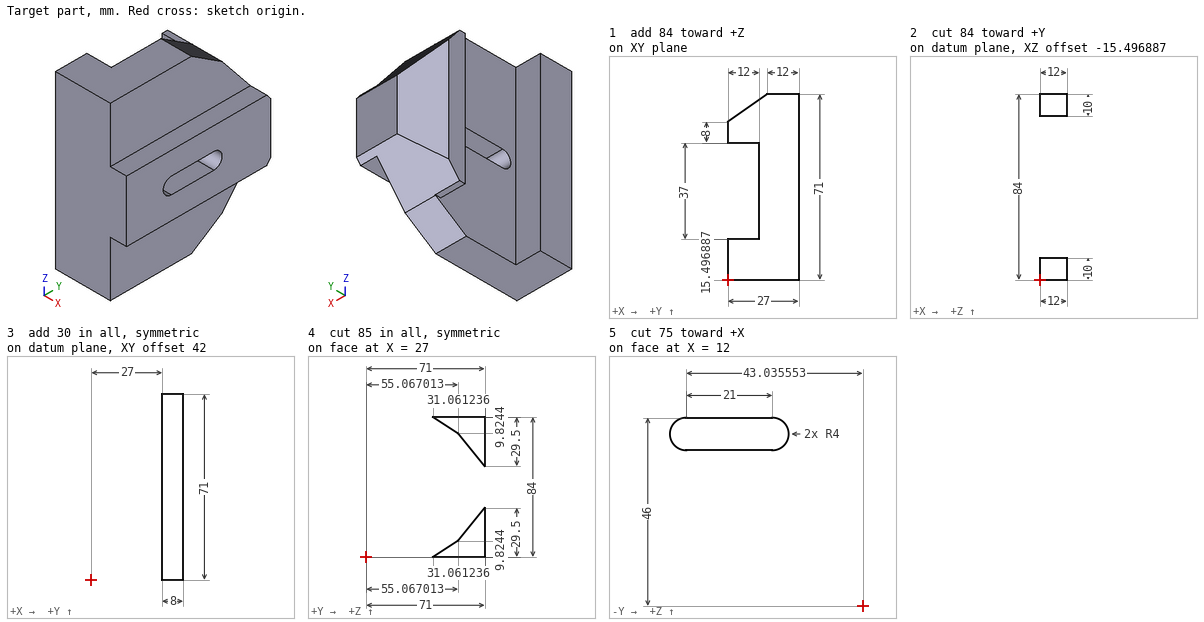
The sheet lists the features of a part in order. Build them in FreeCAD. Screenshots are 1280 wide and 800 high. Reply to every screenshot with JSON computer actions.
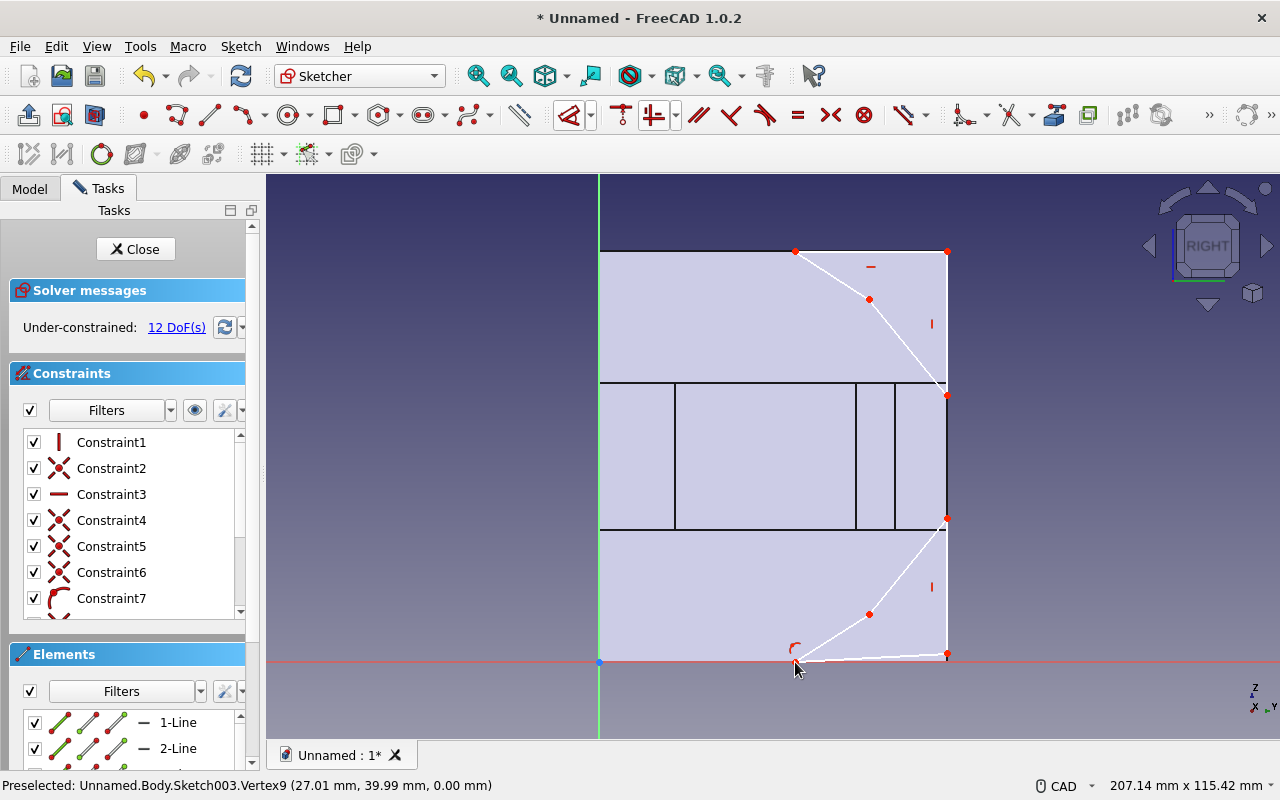
{"action": "left_click", "coordinate": [841, 660]}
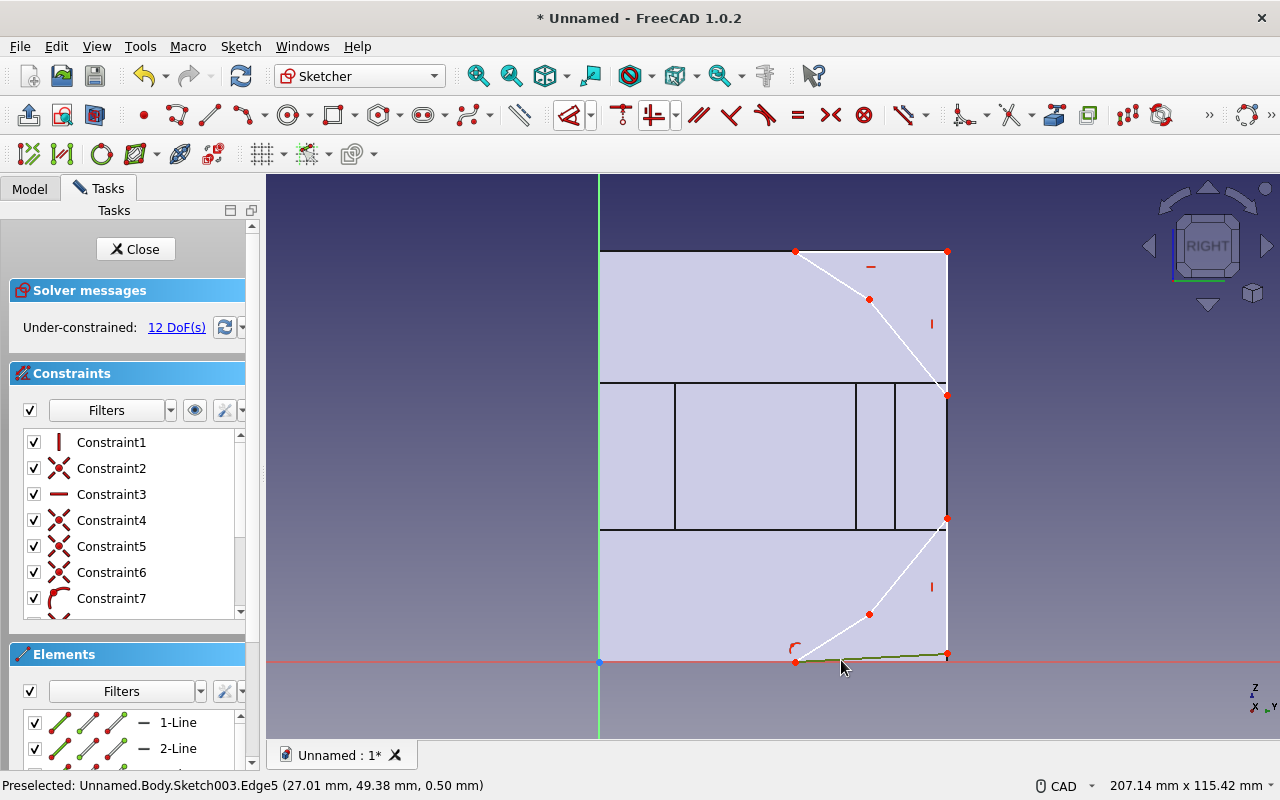
{"action": "left_click", "coordinate": [676, 116]}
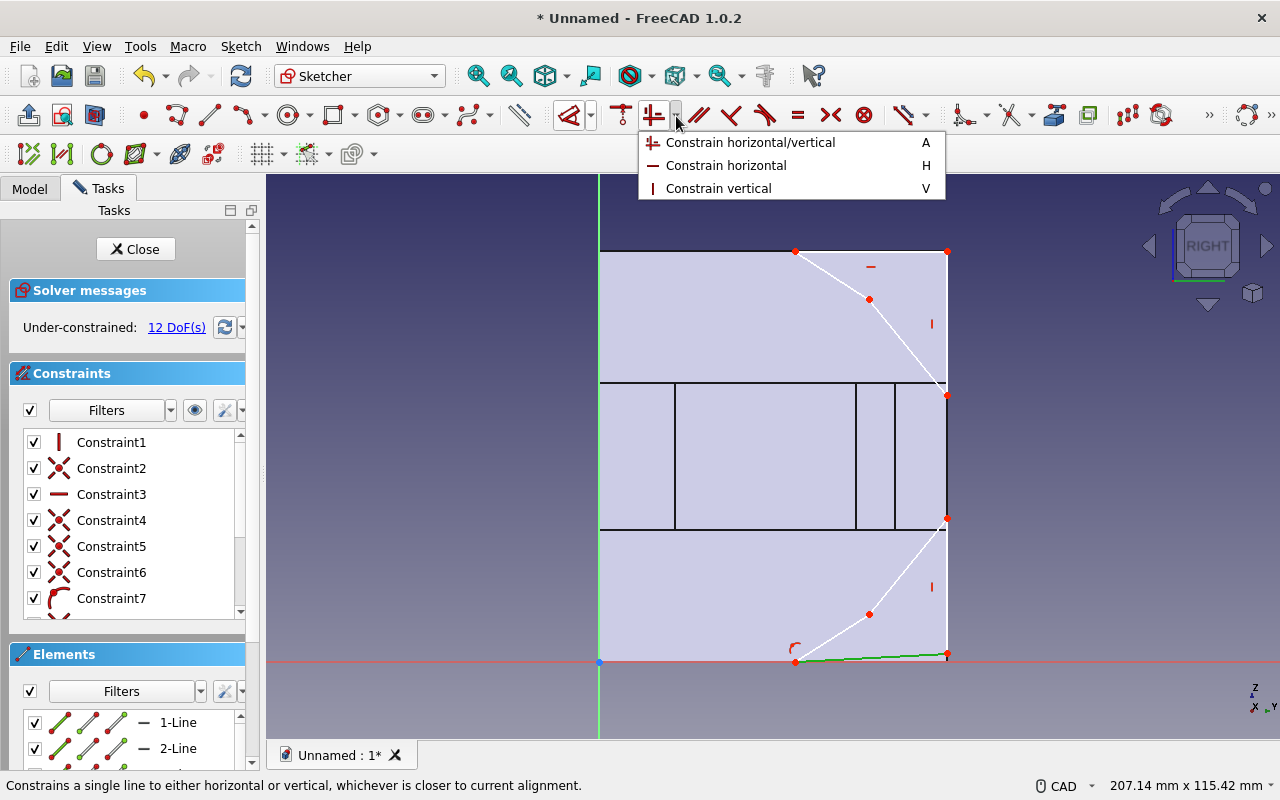
{"action": "left_click", "coordinate": [792, 166]}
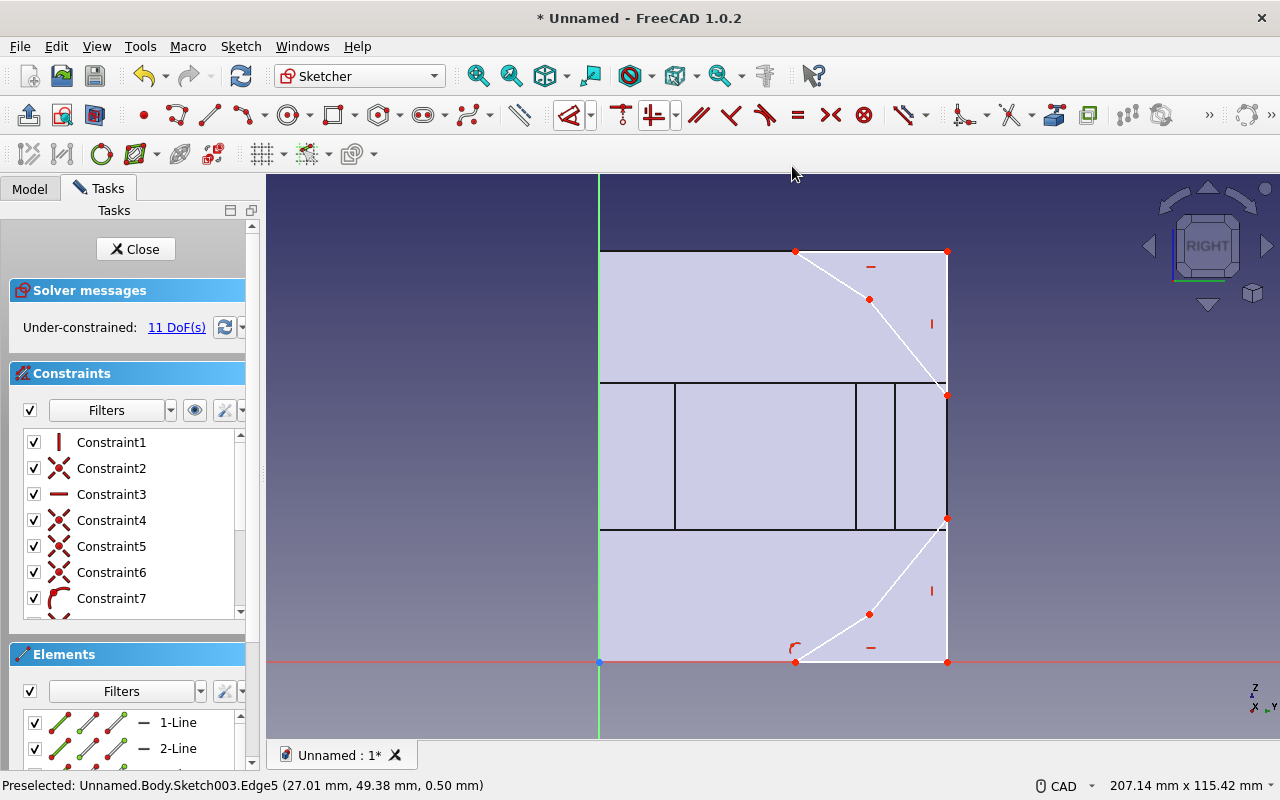
{"action": "left_click", "coordinate": [947, 396]}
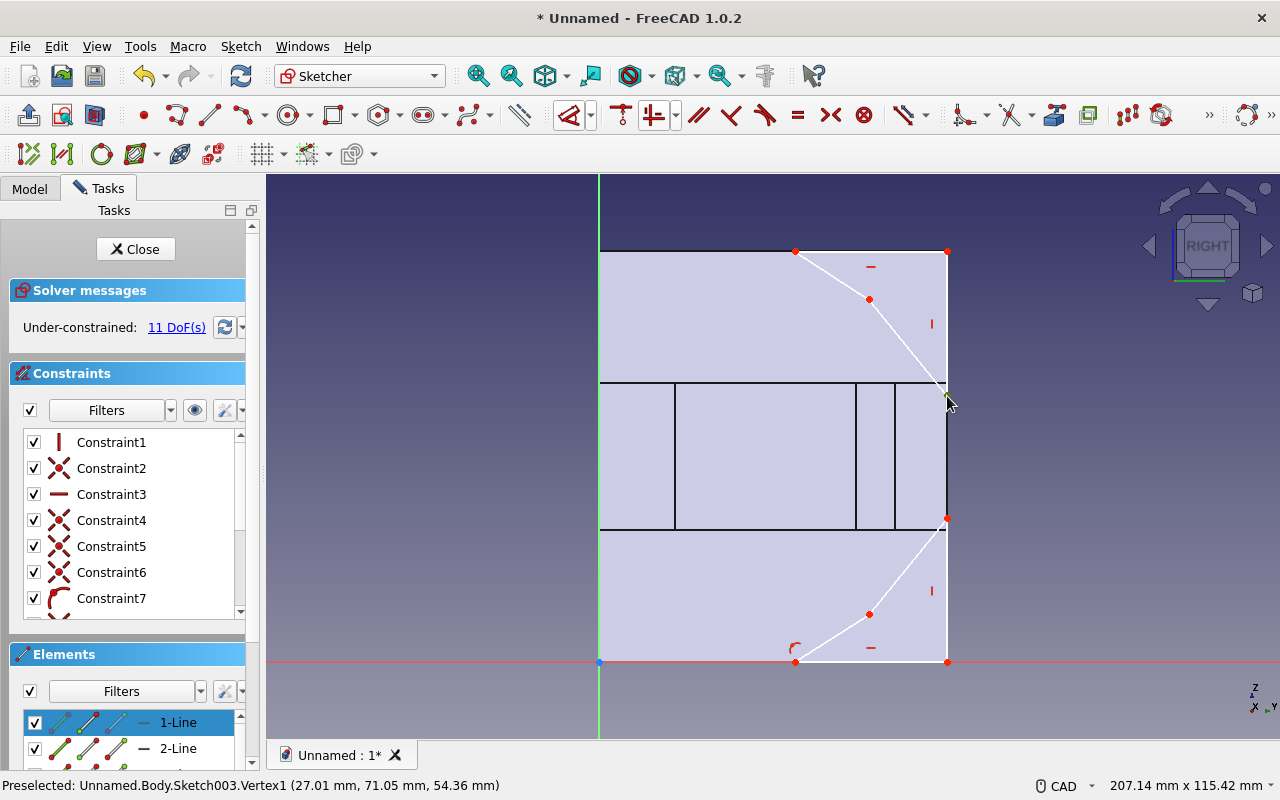
{"action": "left_click", "coordinate": [590, 116]}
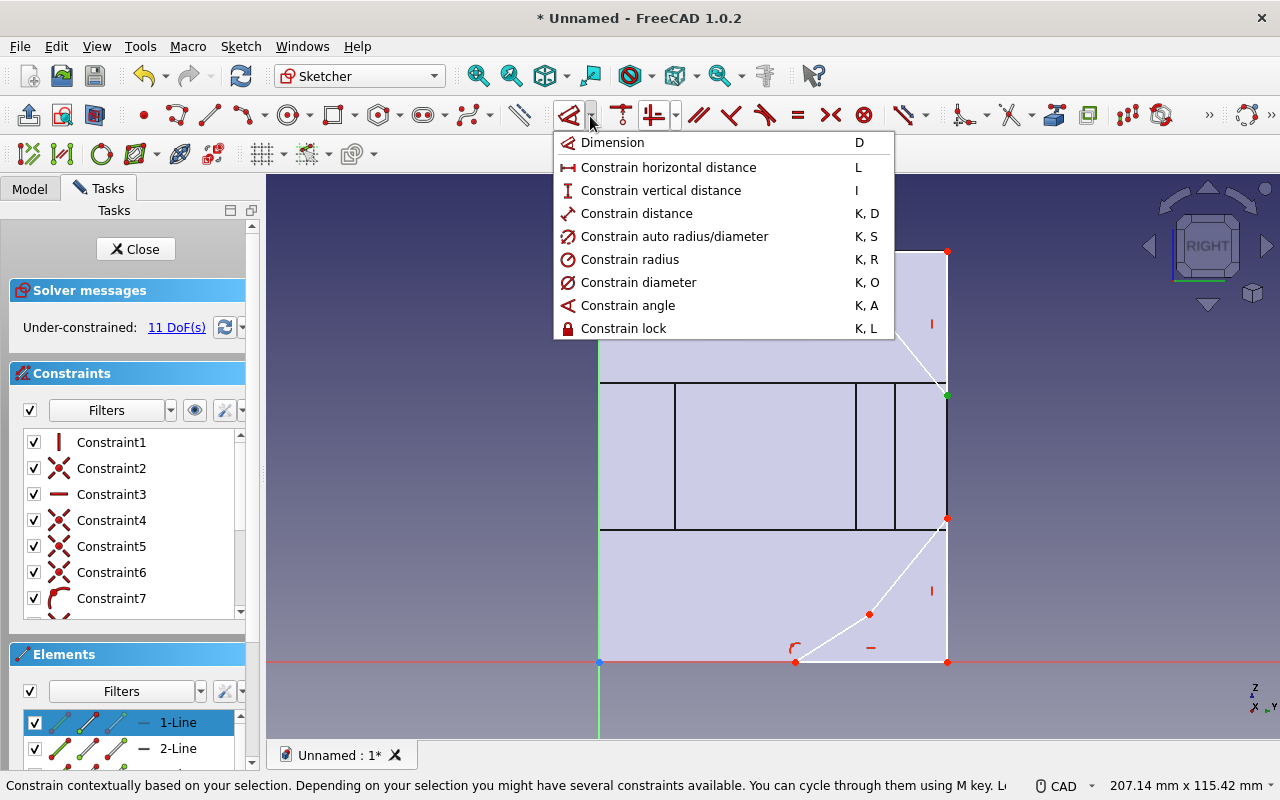
{"action": "left_click", "coordinate": [724, 168]}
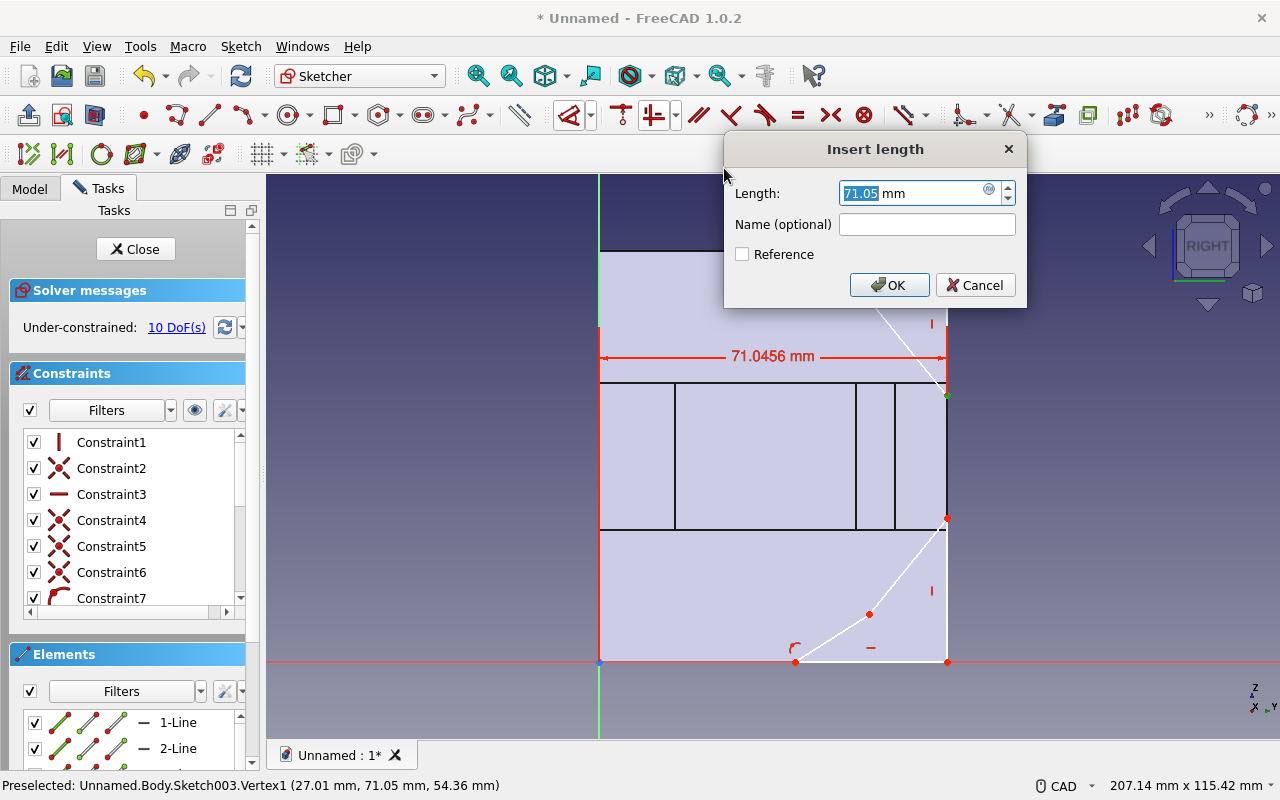
{"action": "type", "text": "71"}
{"action": "key", "text": "Return"}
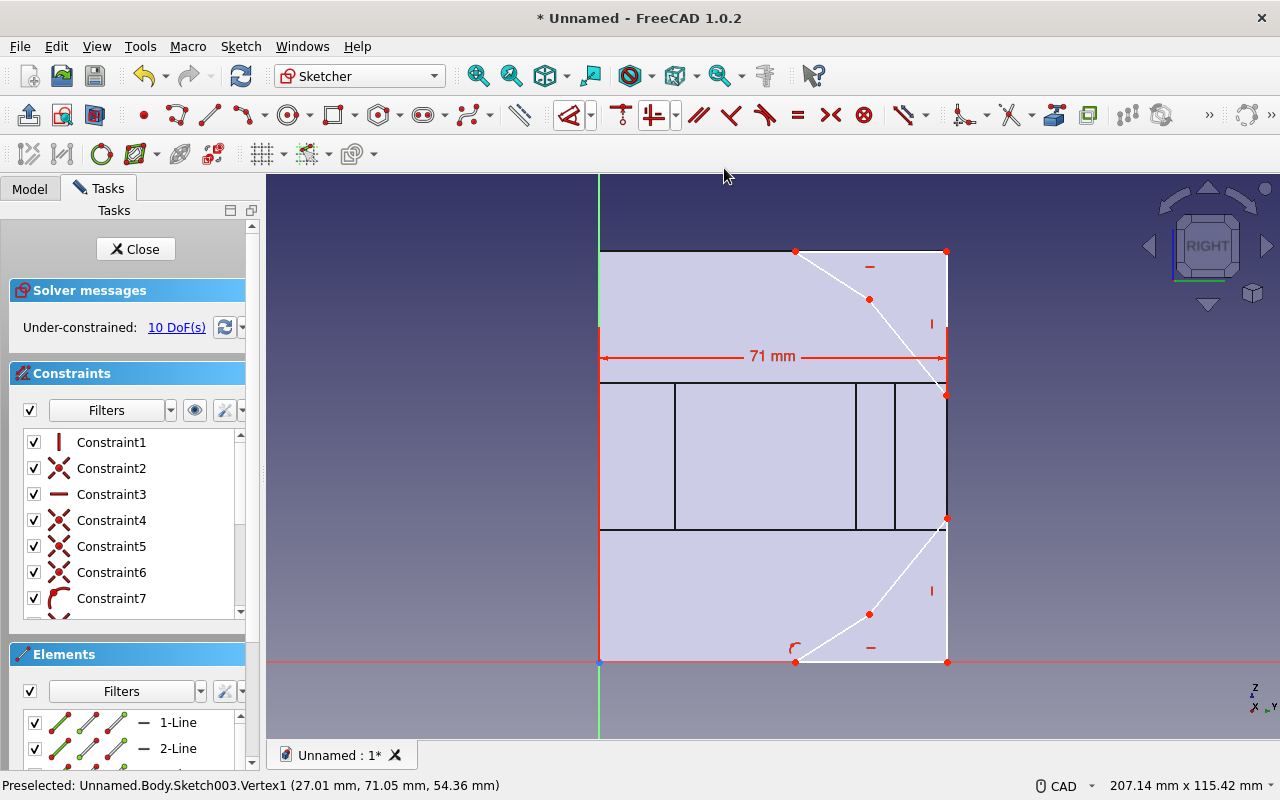
{"action": "left_click", "coordinate": [947, 252]}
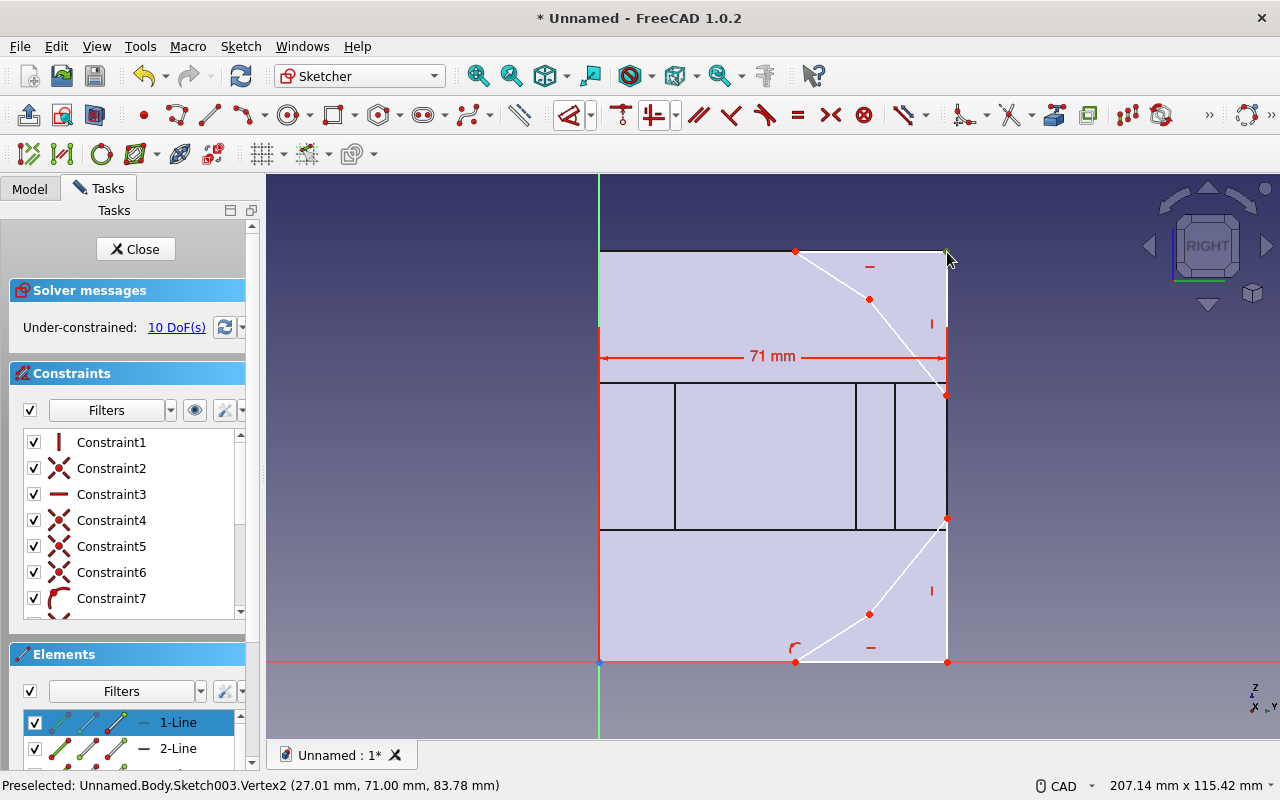
{"action": "left_click", "coordinate": [590, 116]}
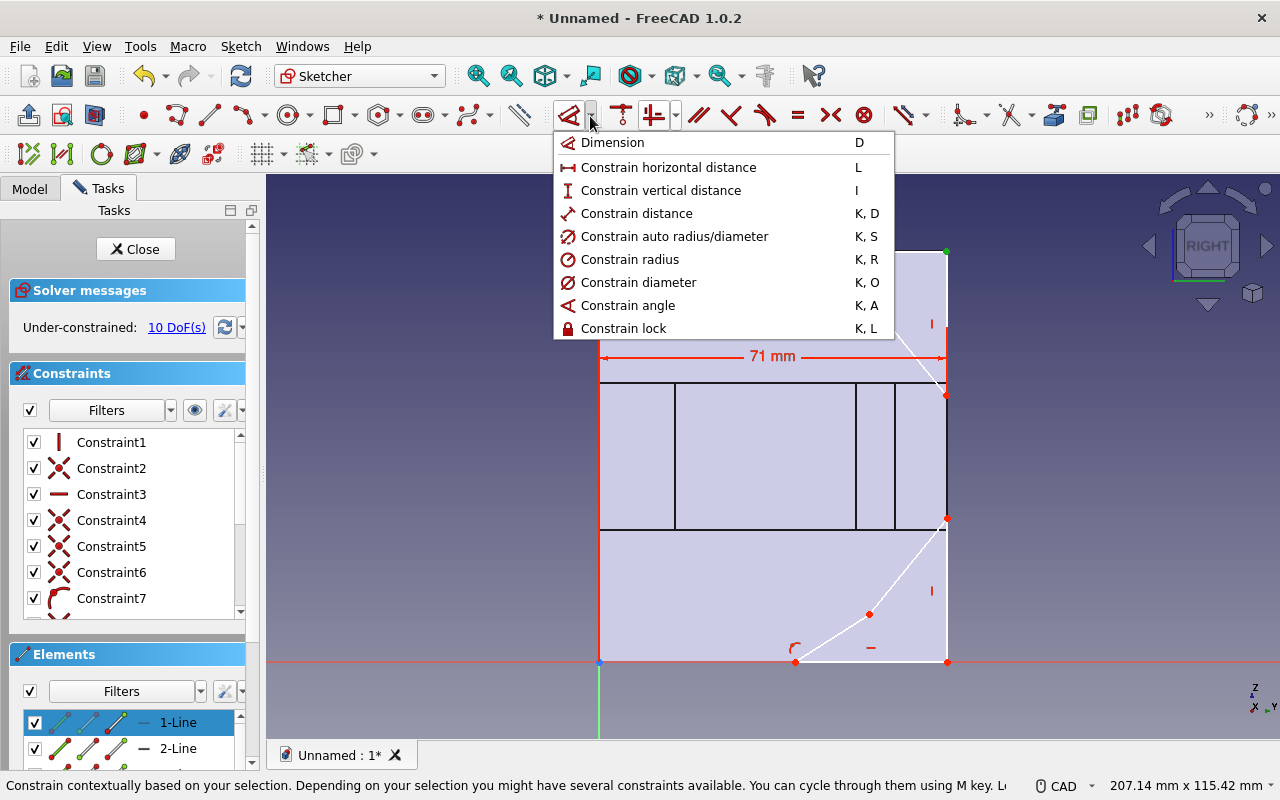
{"action": "left_click", "coordinate": [724, 190]}